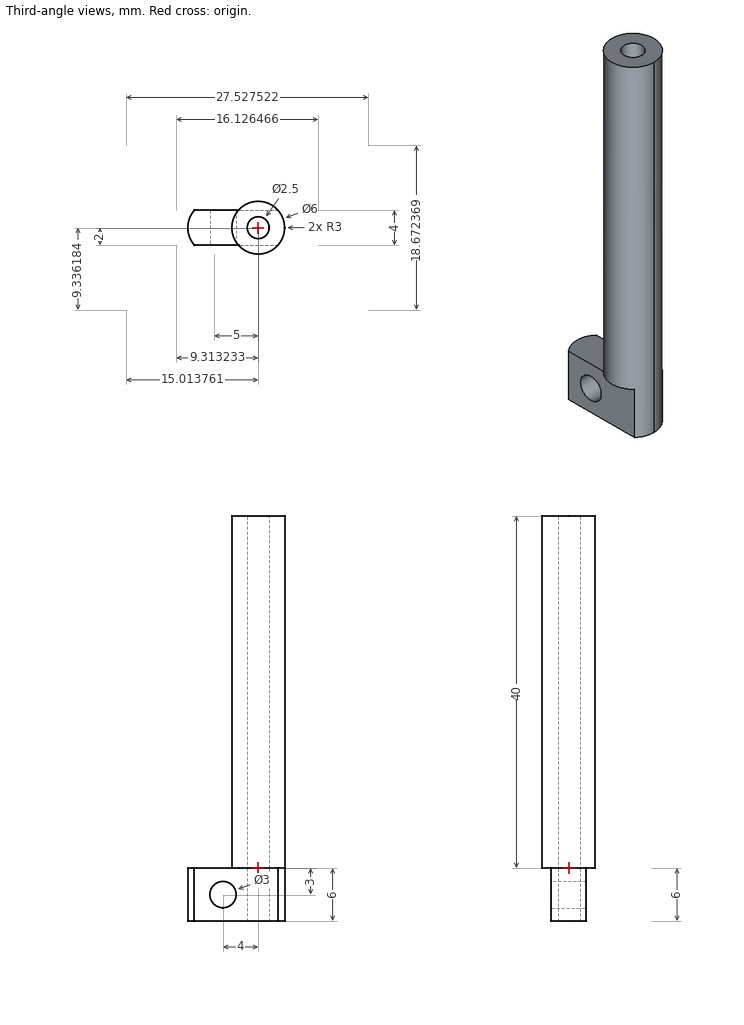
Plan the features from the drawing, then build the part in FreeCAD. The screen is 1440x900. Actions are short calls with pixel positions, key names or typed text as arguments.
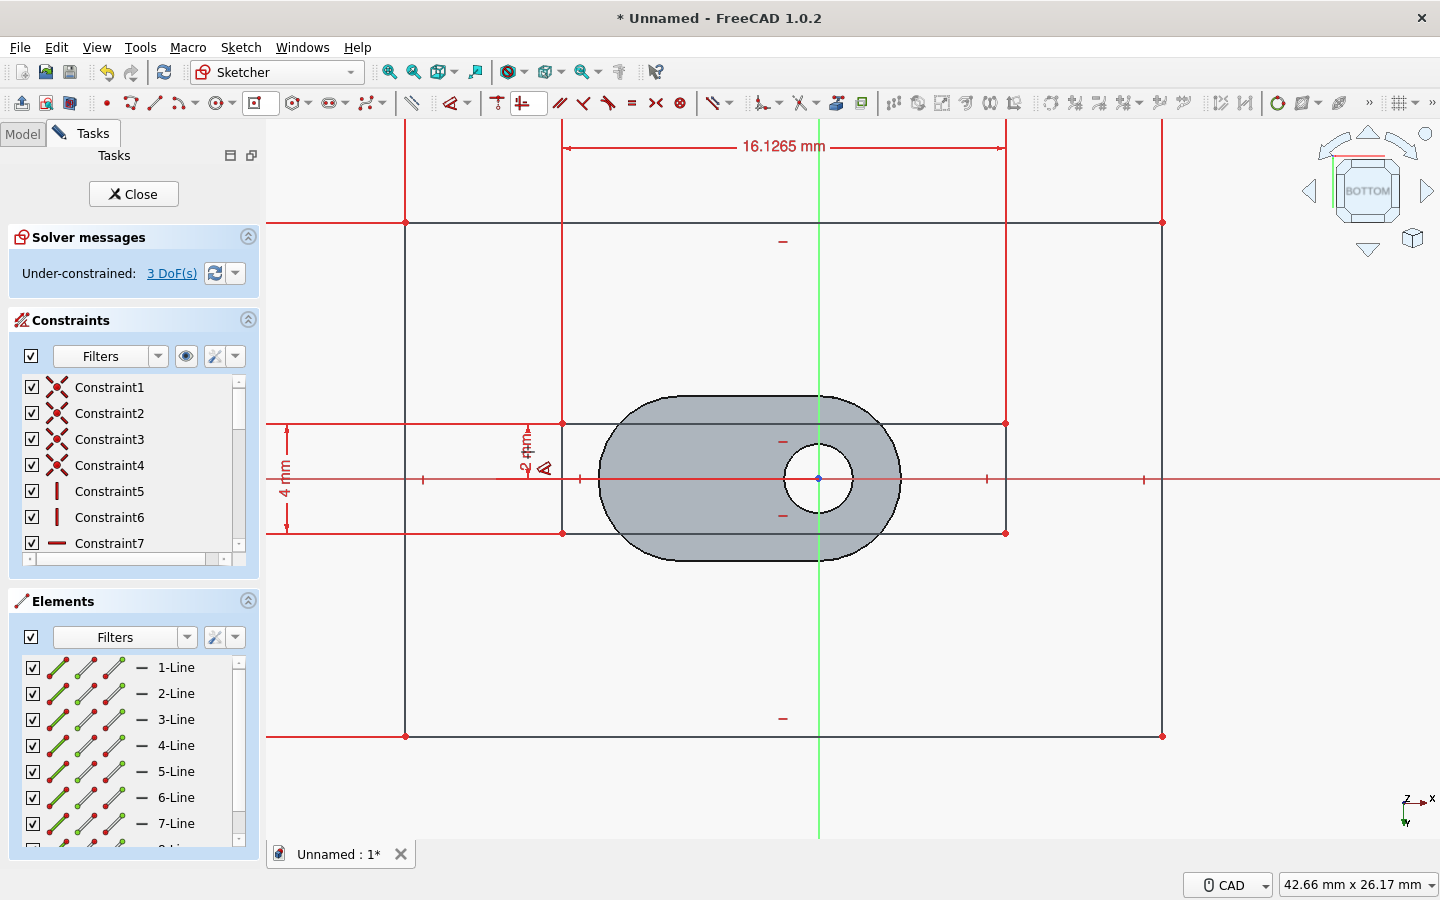
click(405, 223)
click(371, 351)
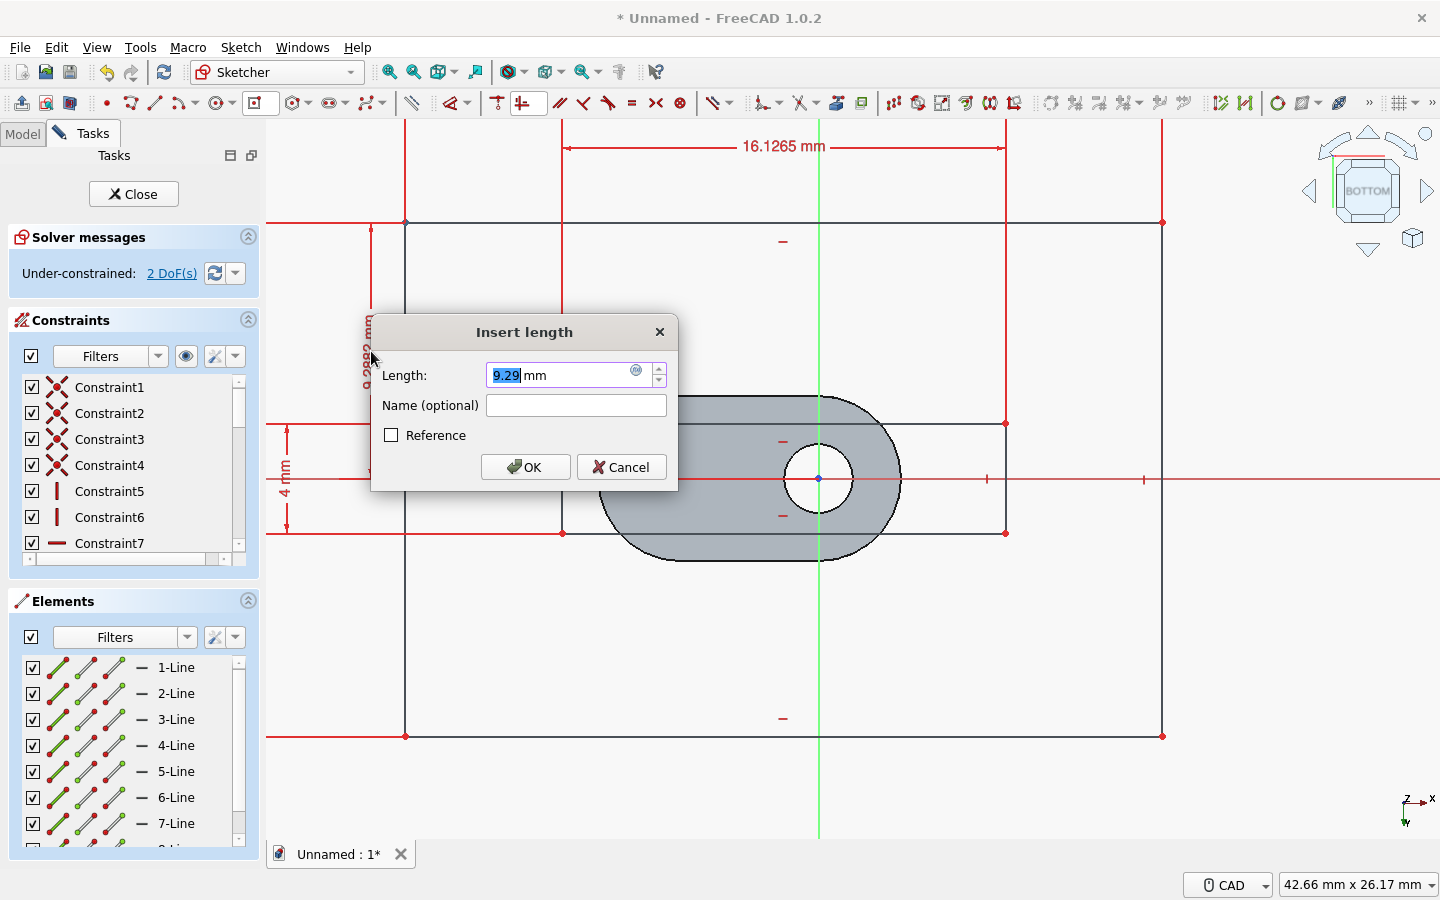
text(9.336184)
key(Return)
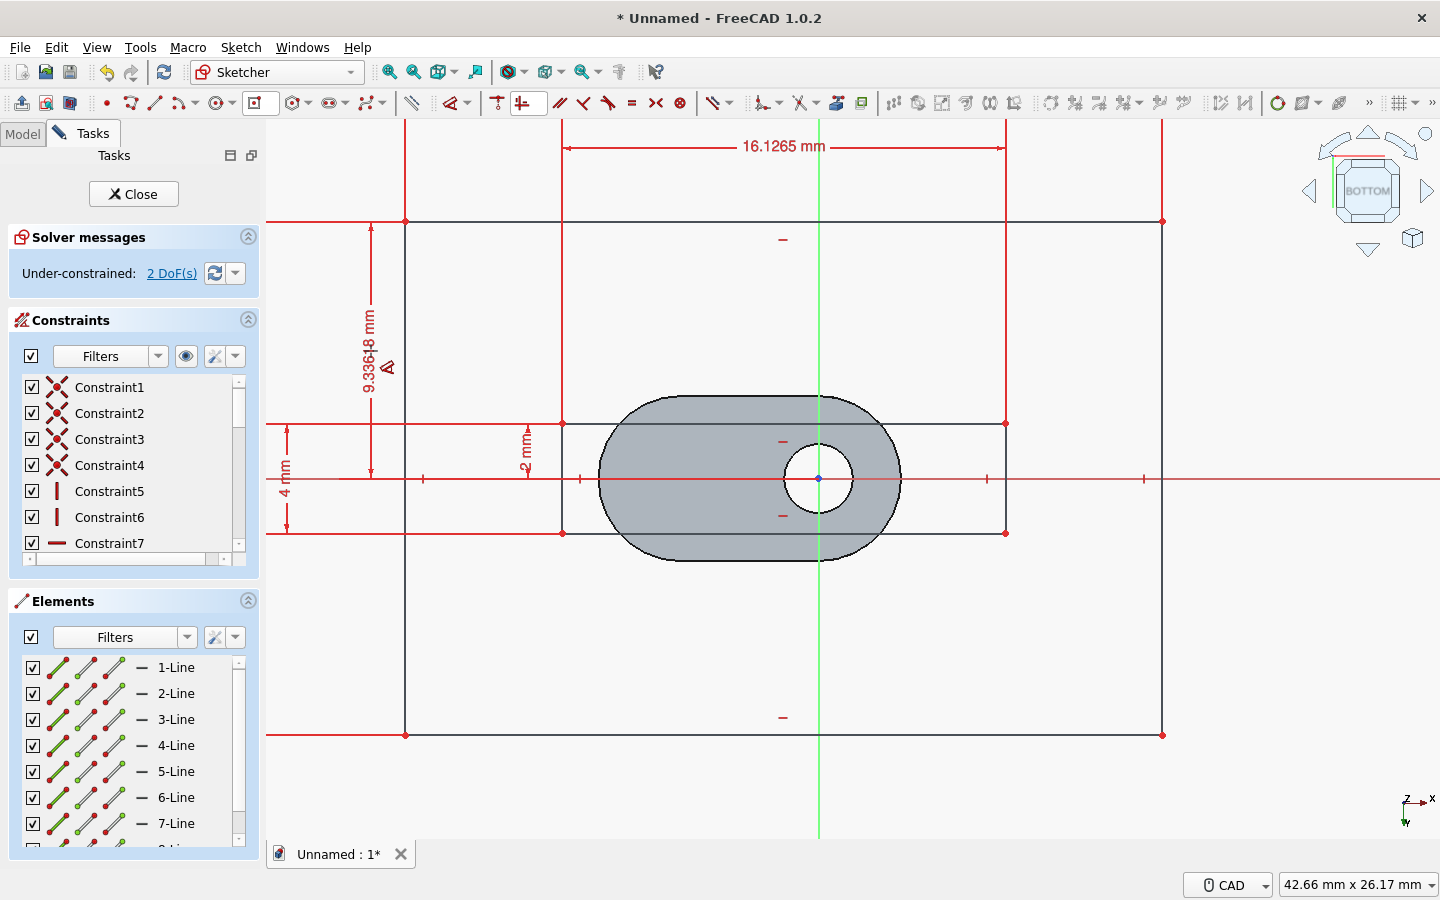
click(562, 424)
click(690, 390)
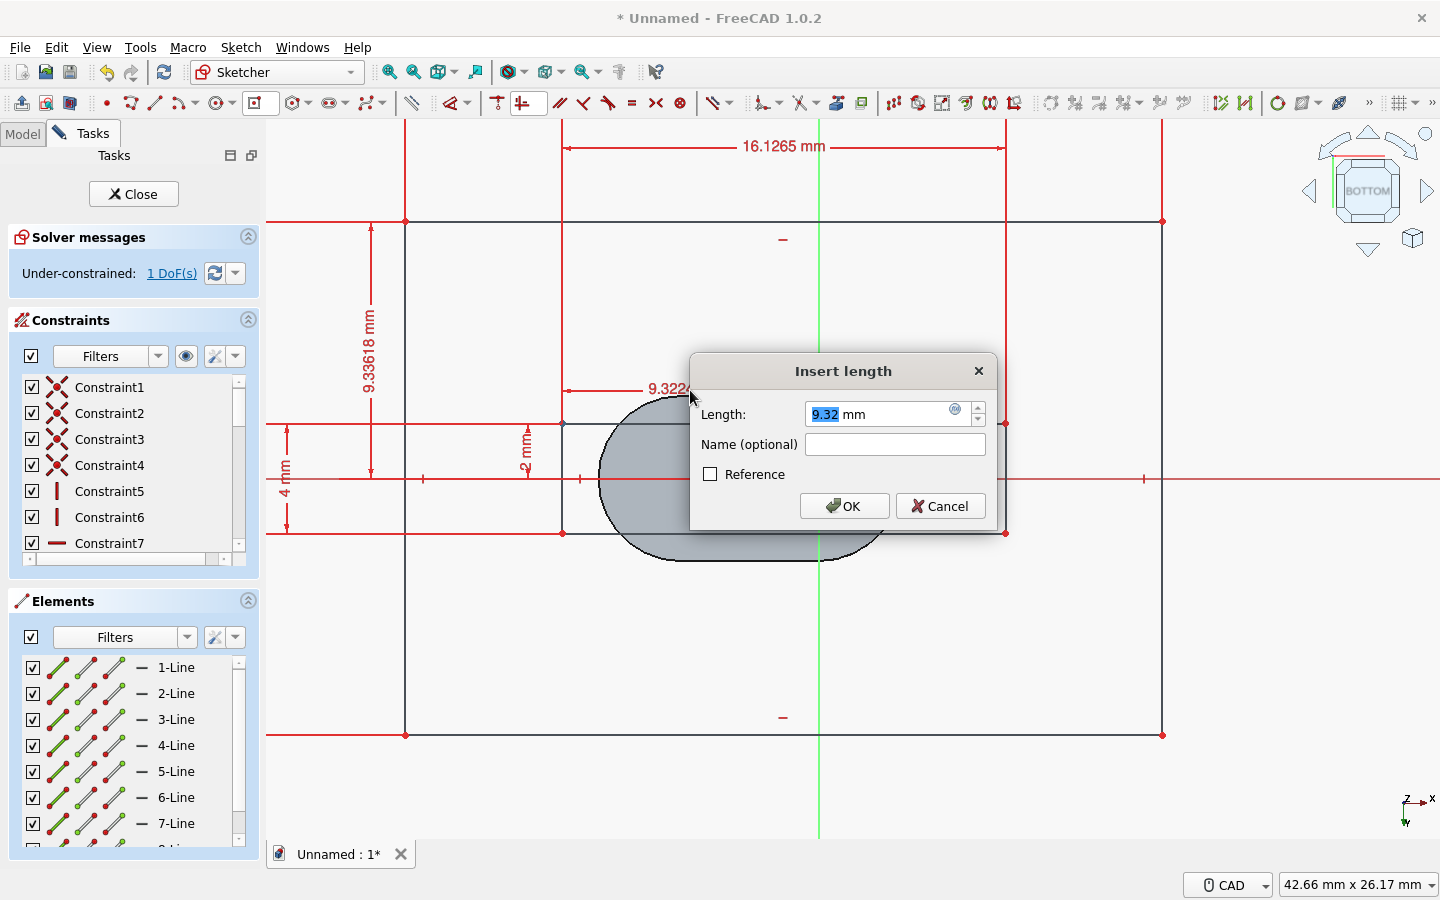
text(9.313233)
key(Return)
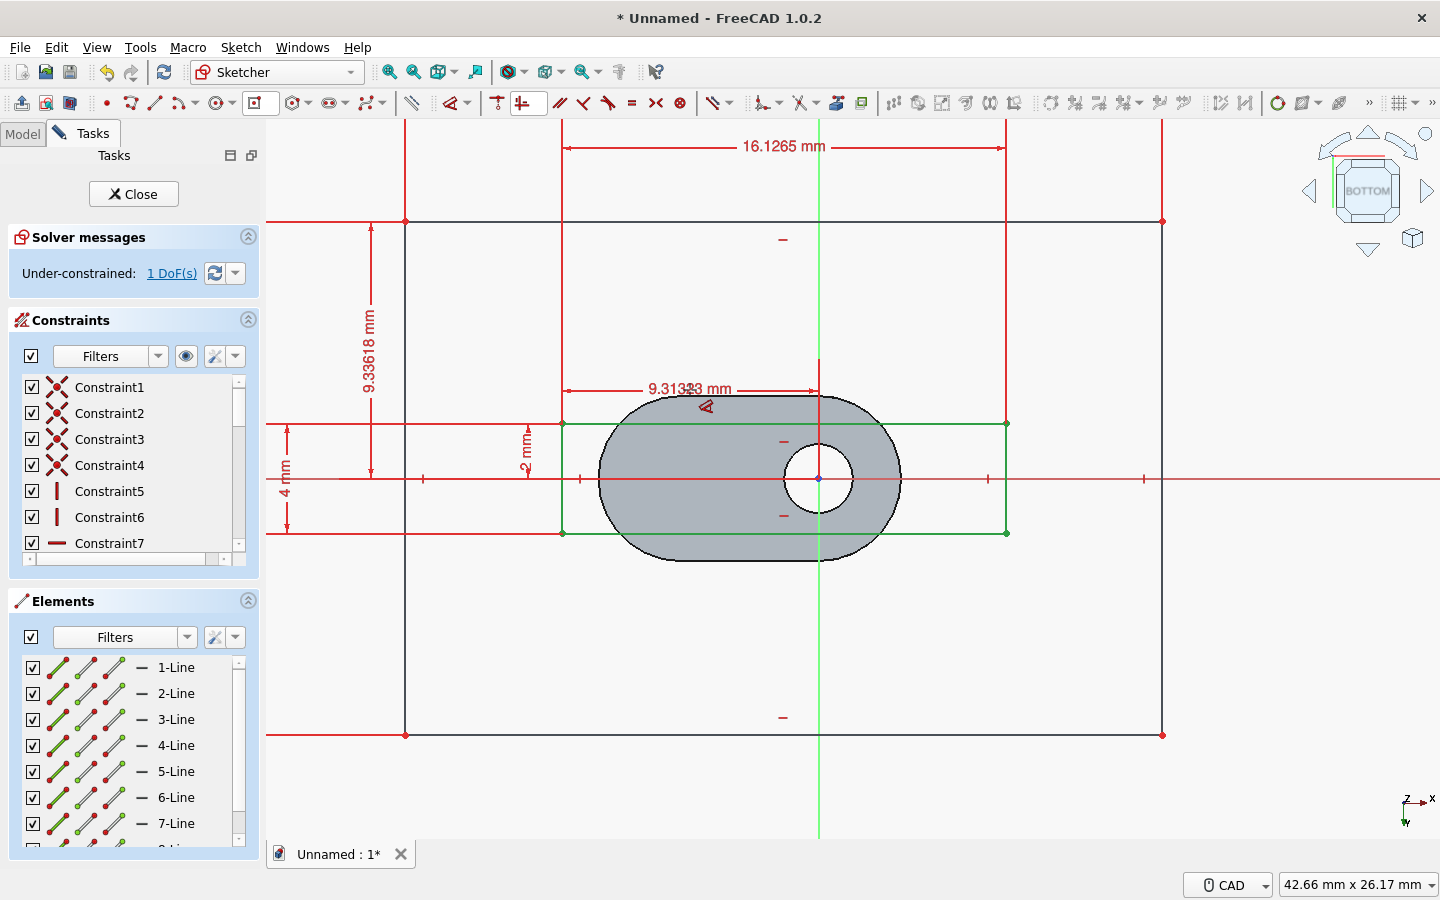
click(405, 222)
click(612, 188)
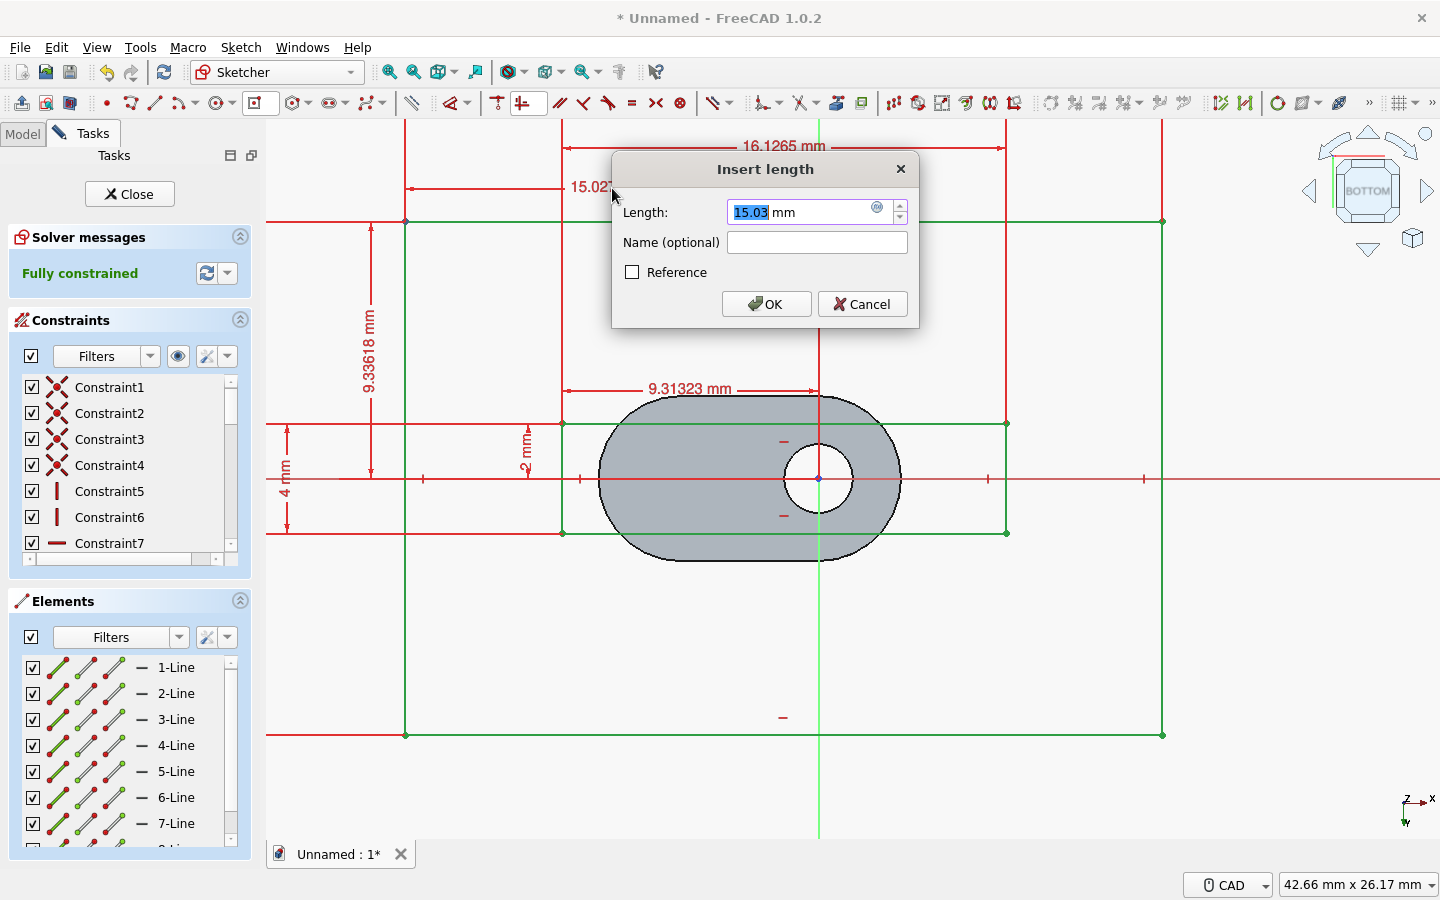
text(15.013761)
key(Return)
key(Escape)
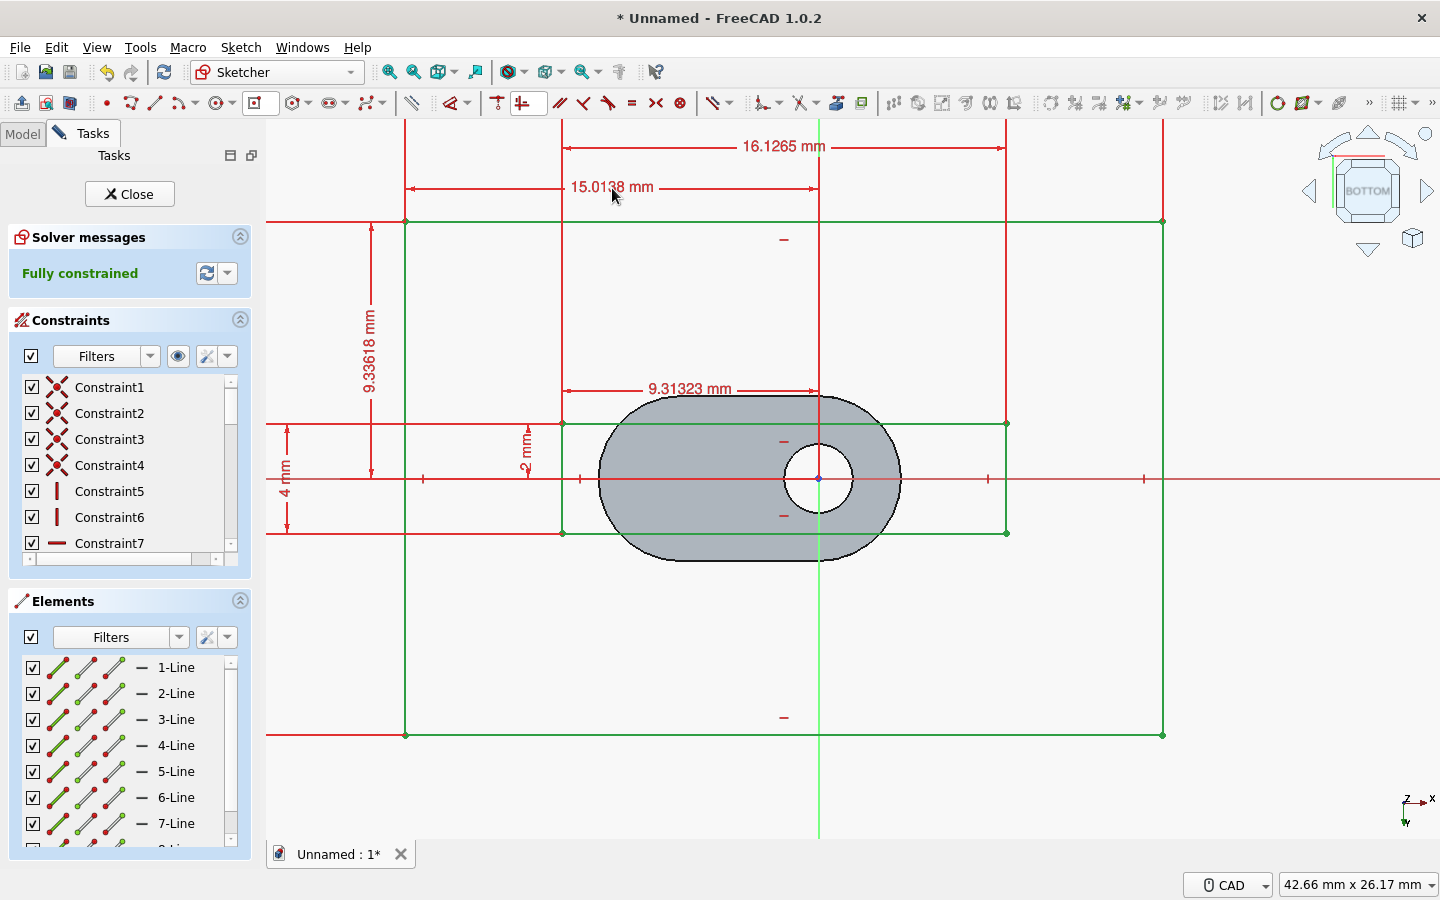
click(130, 194)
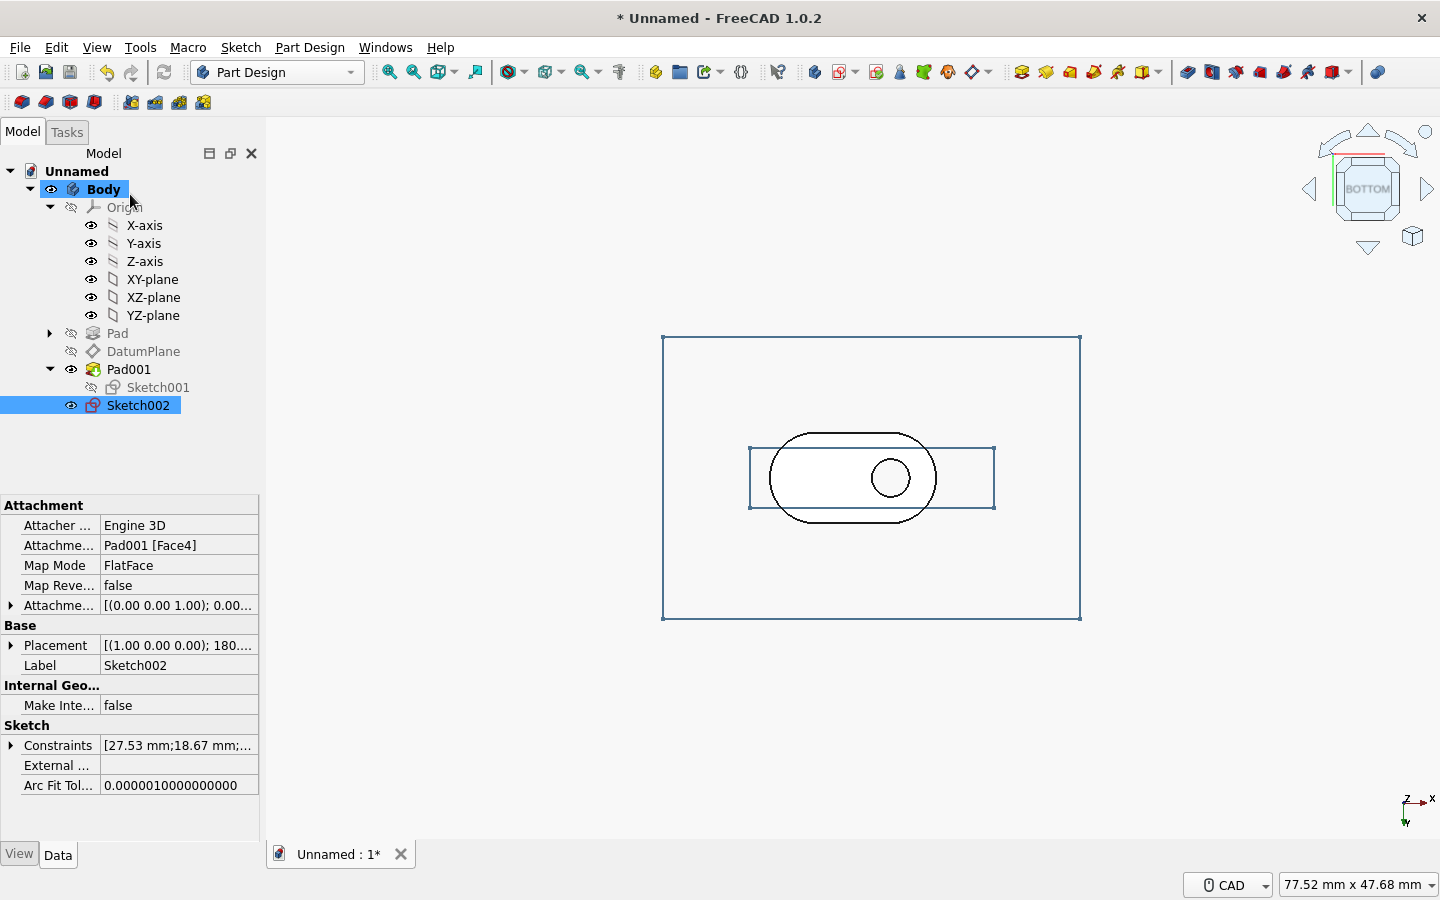
click(1188, 72)